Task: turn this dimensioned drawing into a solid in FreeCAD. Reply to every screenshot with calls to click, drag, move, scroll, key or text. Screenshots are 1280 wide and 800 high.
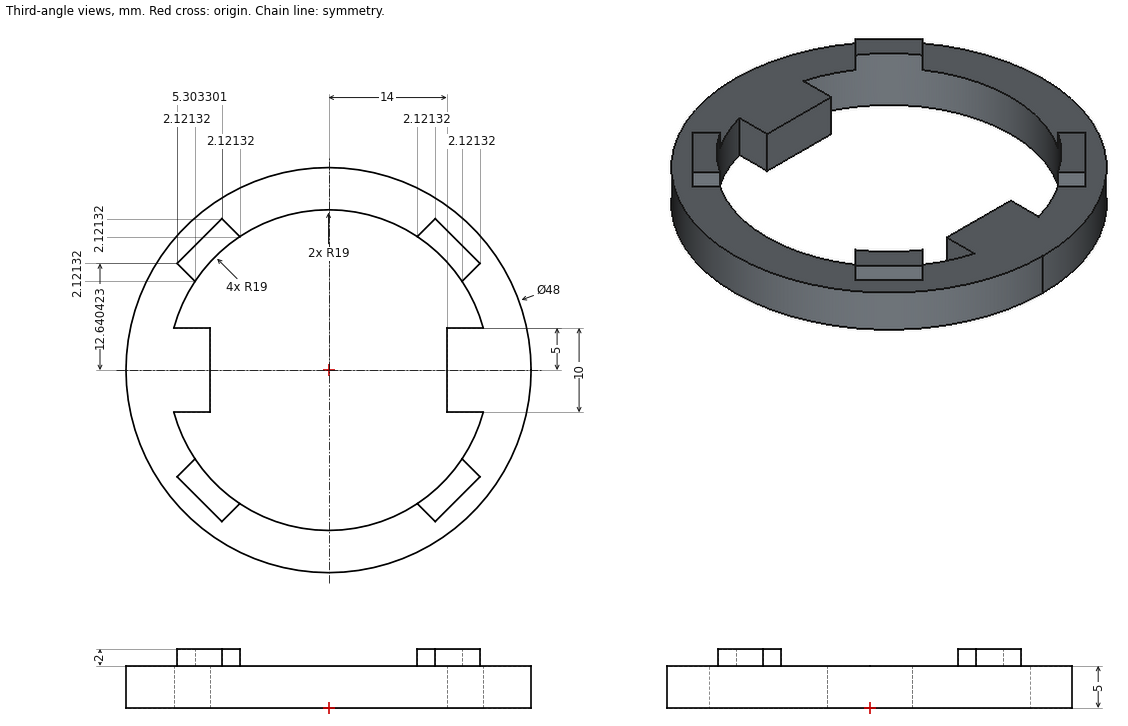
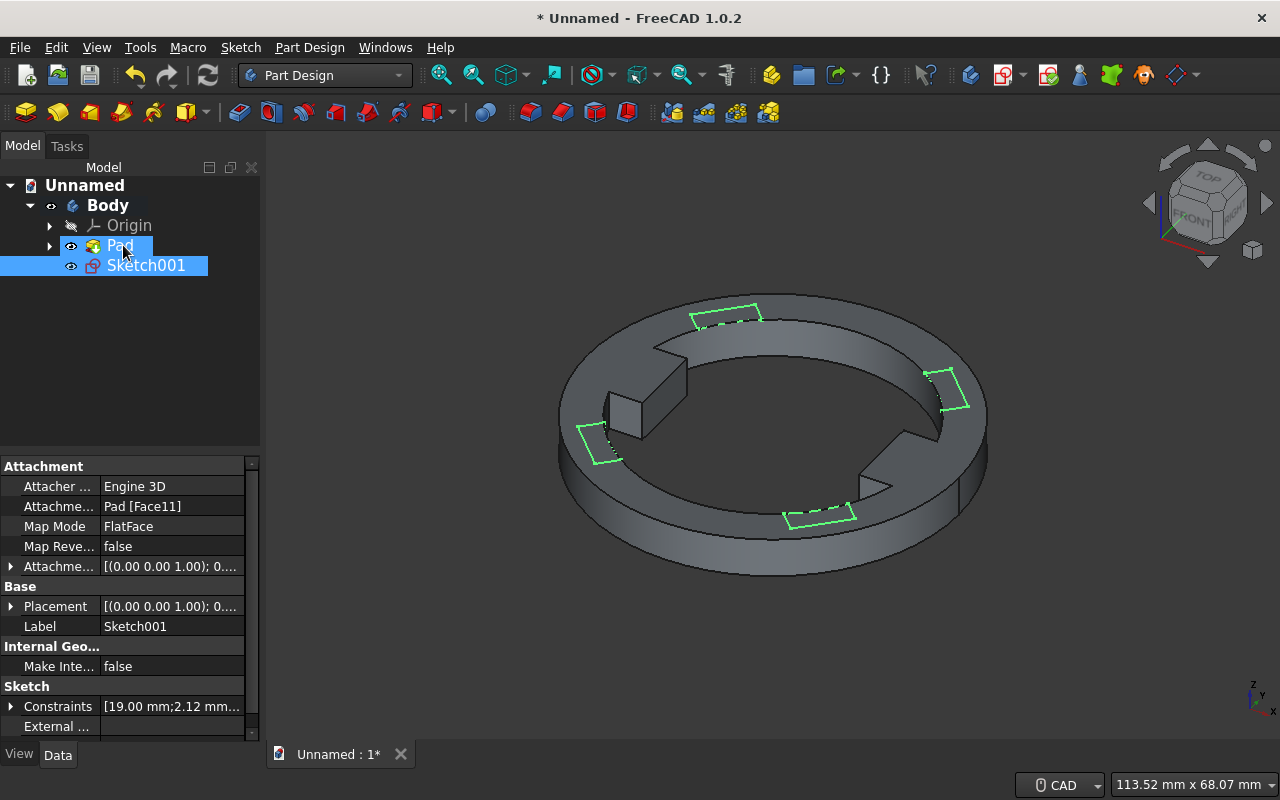
click(26, 112)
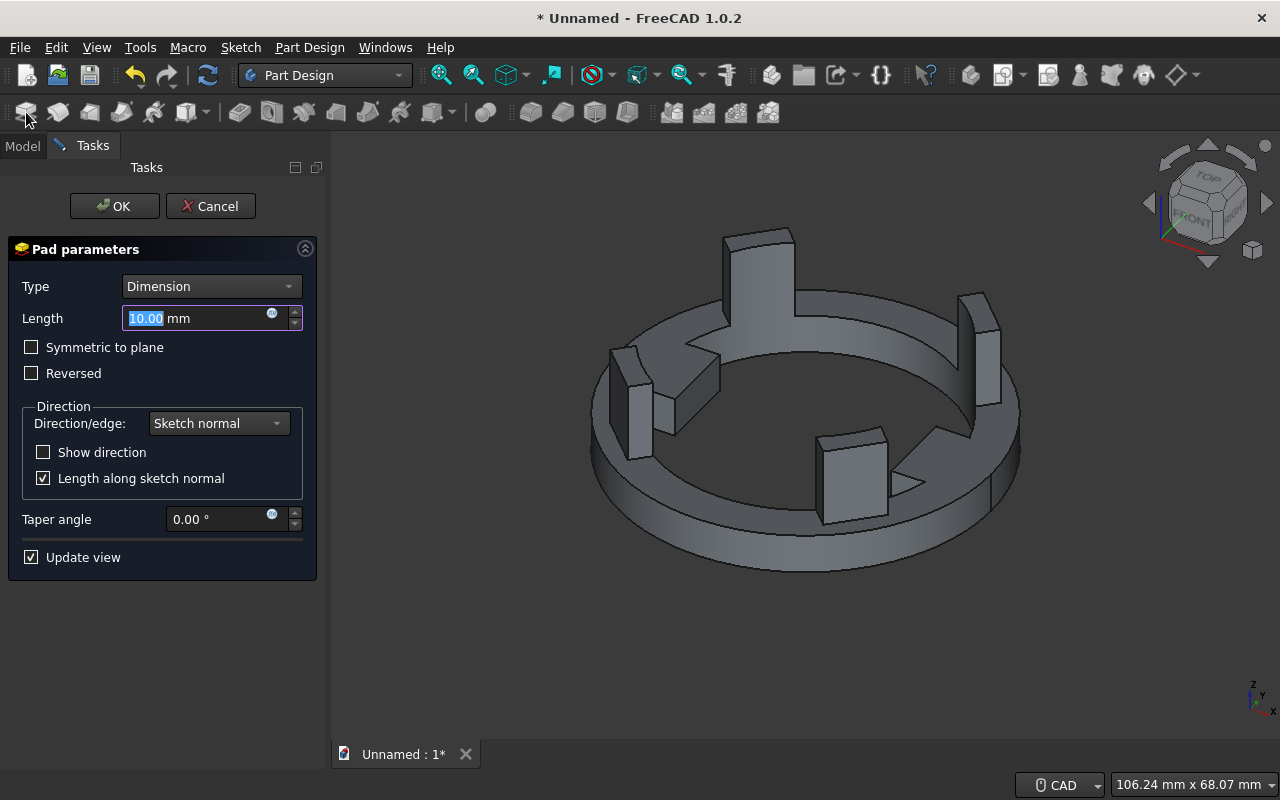
text(2)
key(Tab)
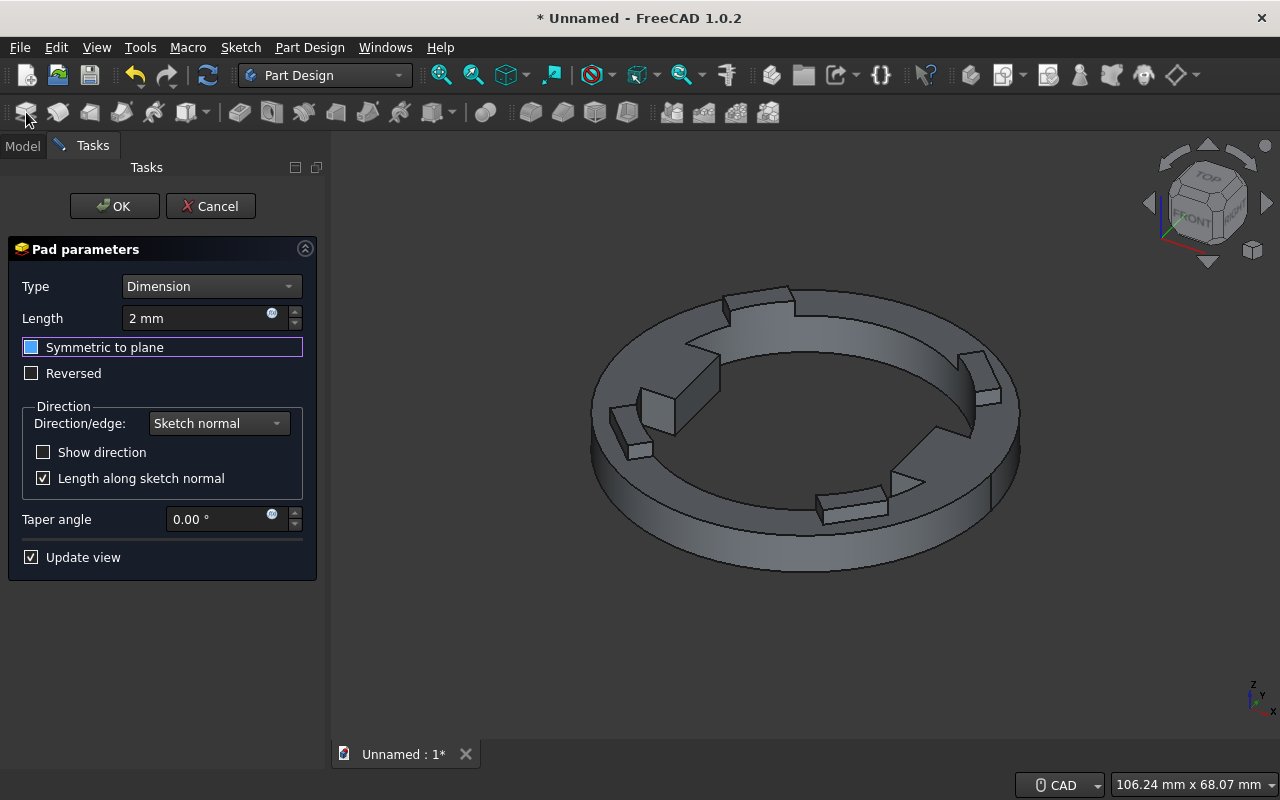
click(115, 206)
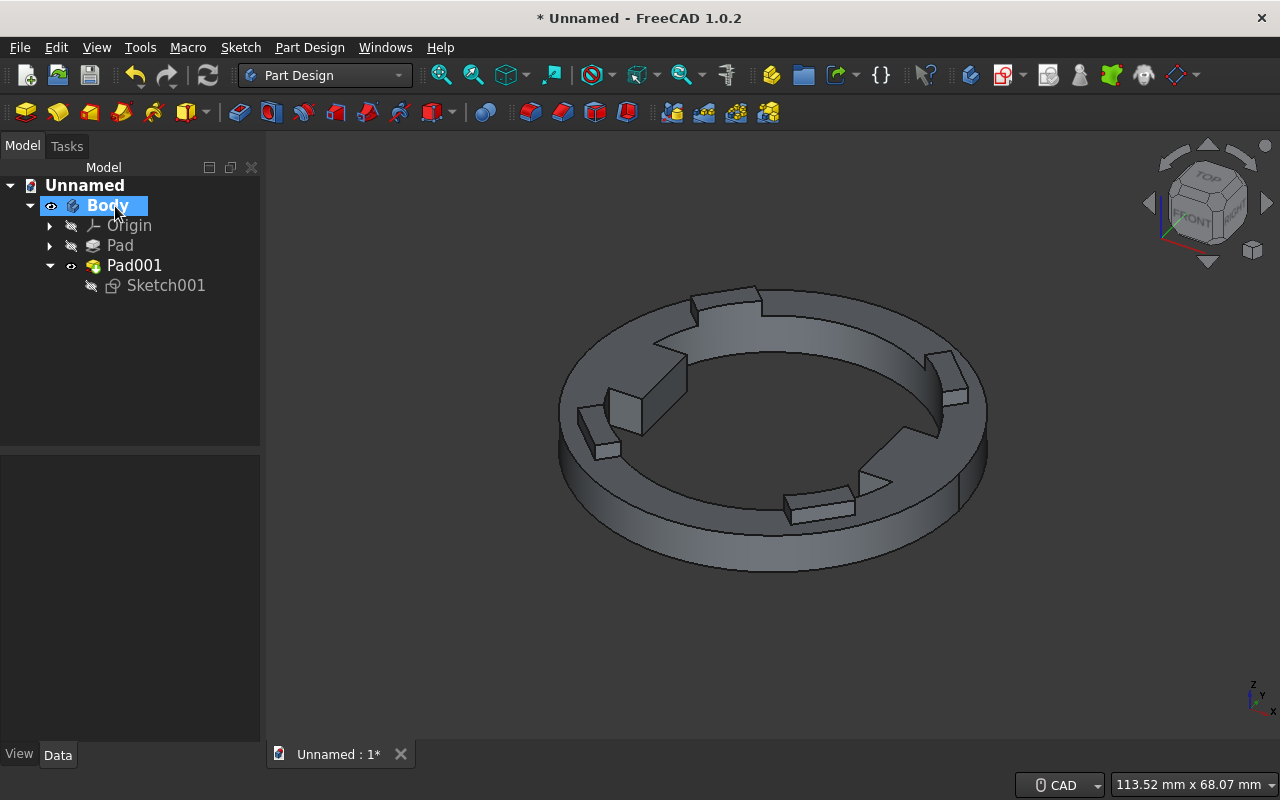
key(0)